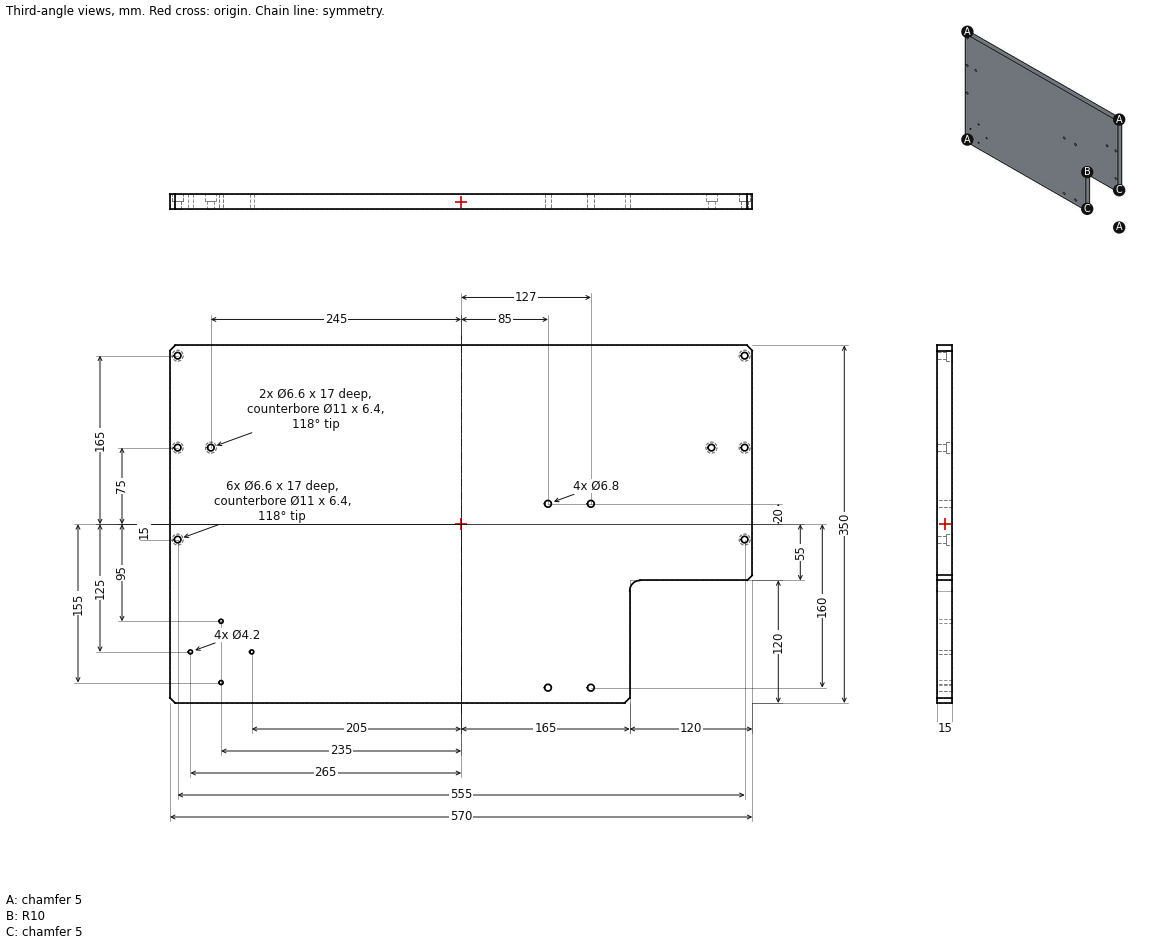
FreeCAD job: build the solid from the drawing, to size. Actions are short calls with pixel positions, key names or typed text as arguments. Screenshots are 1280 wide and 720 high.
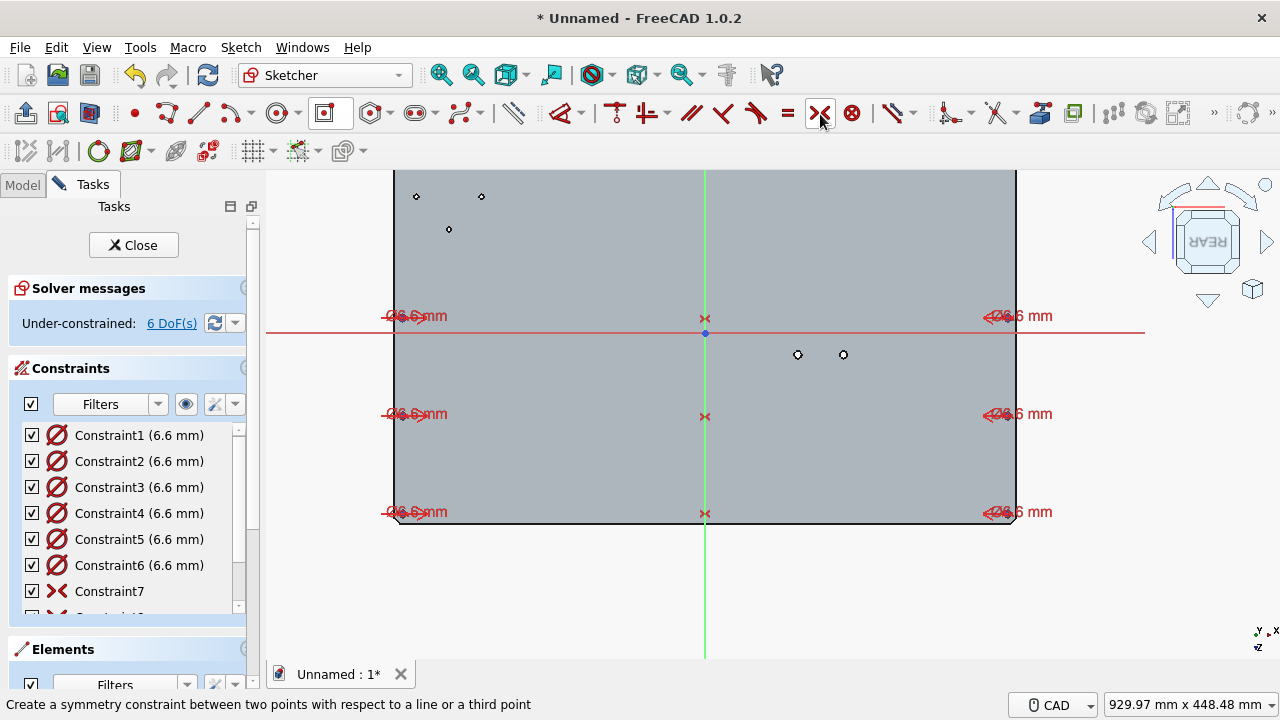
click(560, 114)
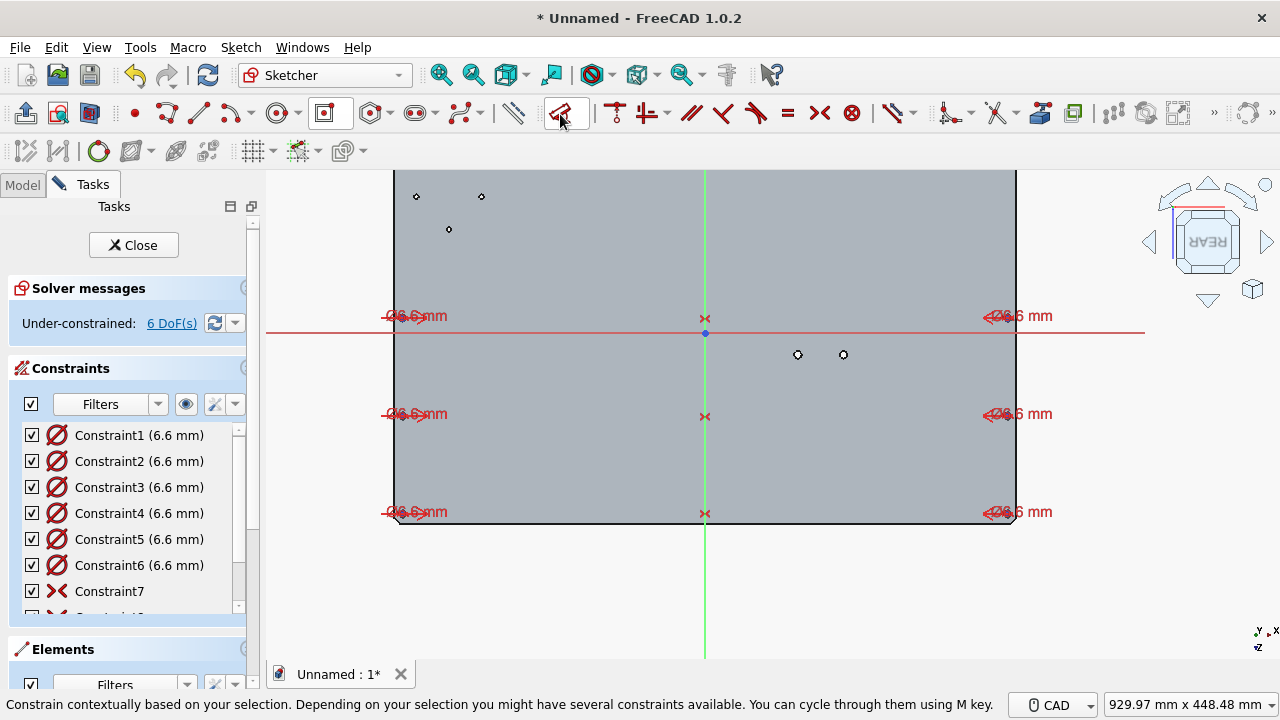
scroll(402, 318, up, 5)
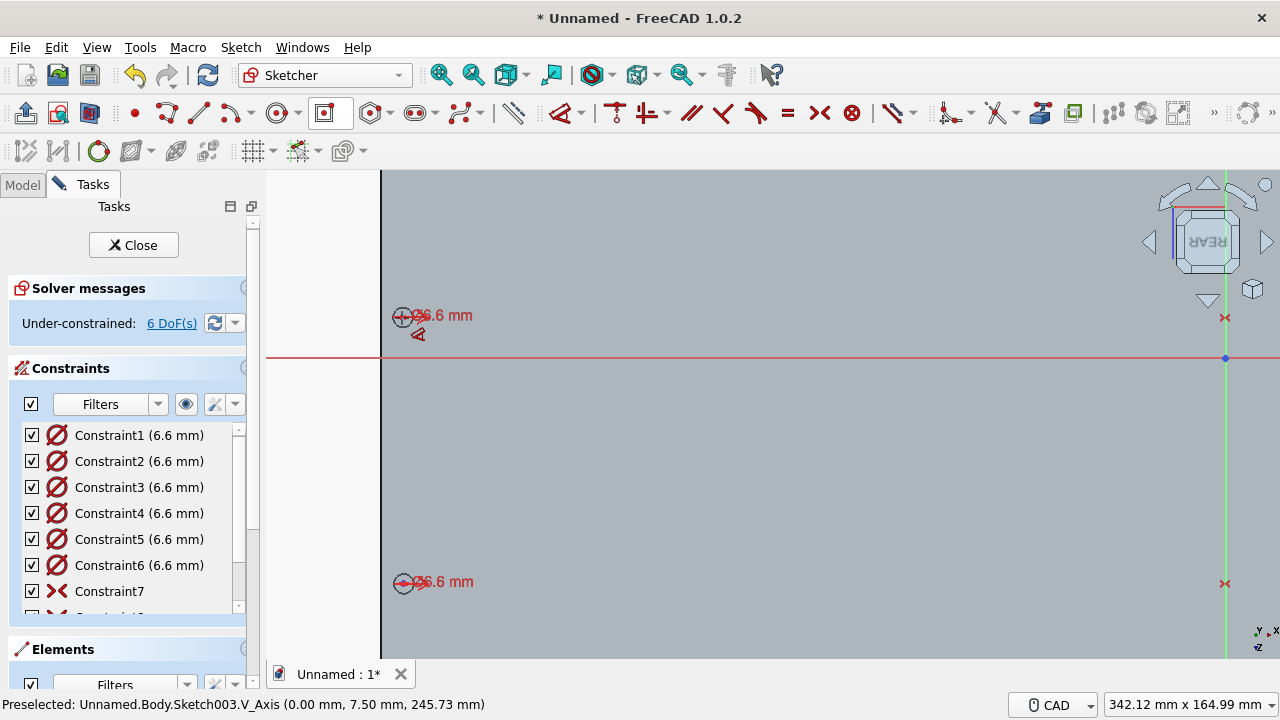
click(403, 317)
click(369, 338)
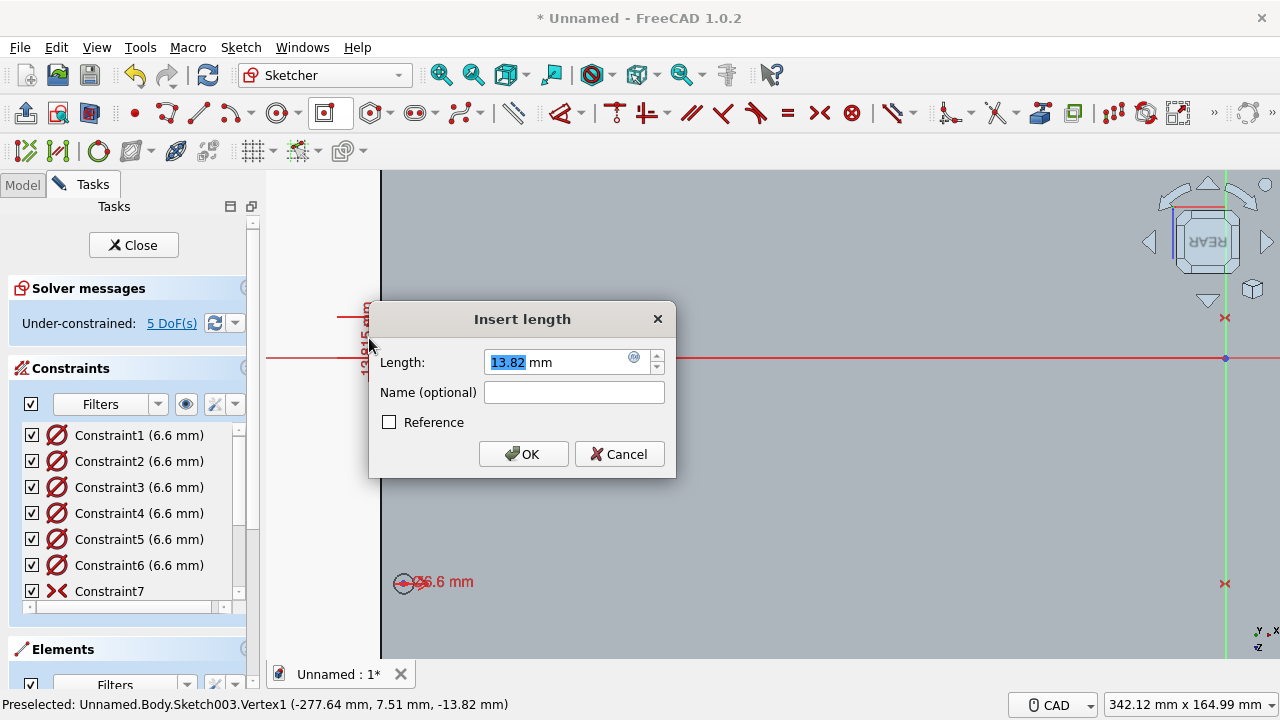
text(15)
key(Return)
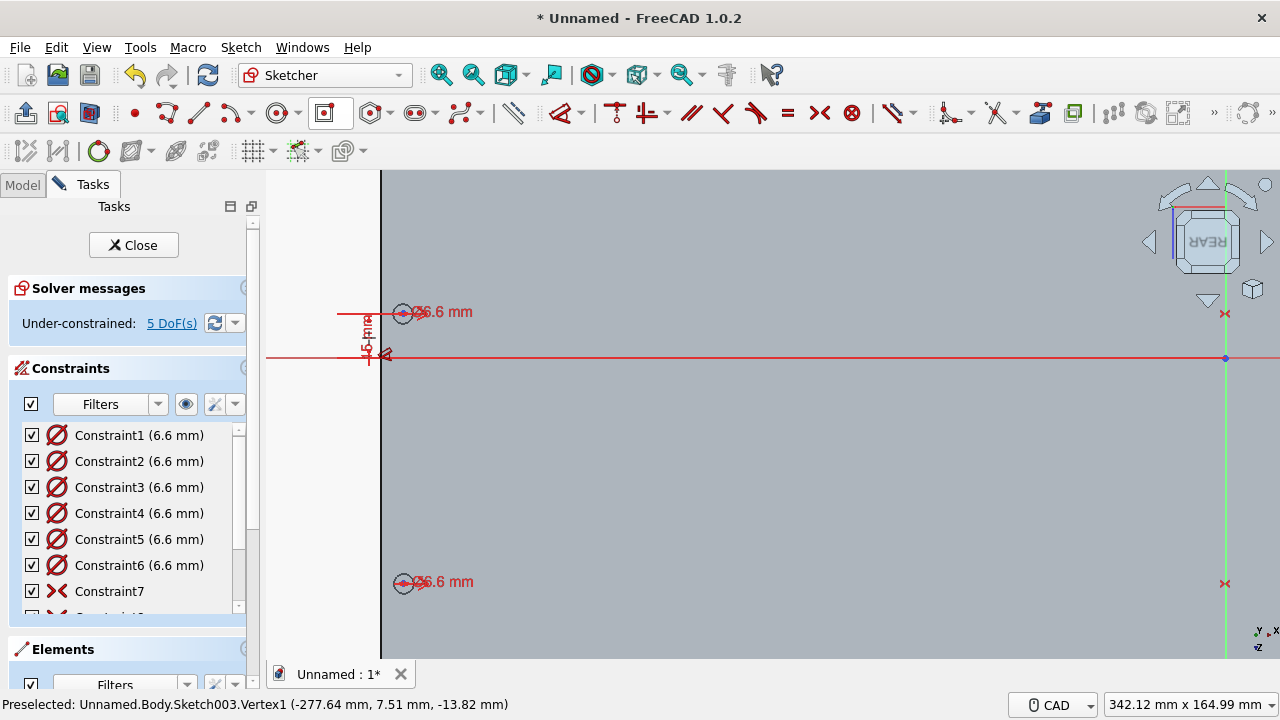
click(404, 584)
click(370, 471)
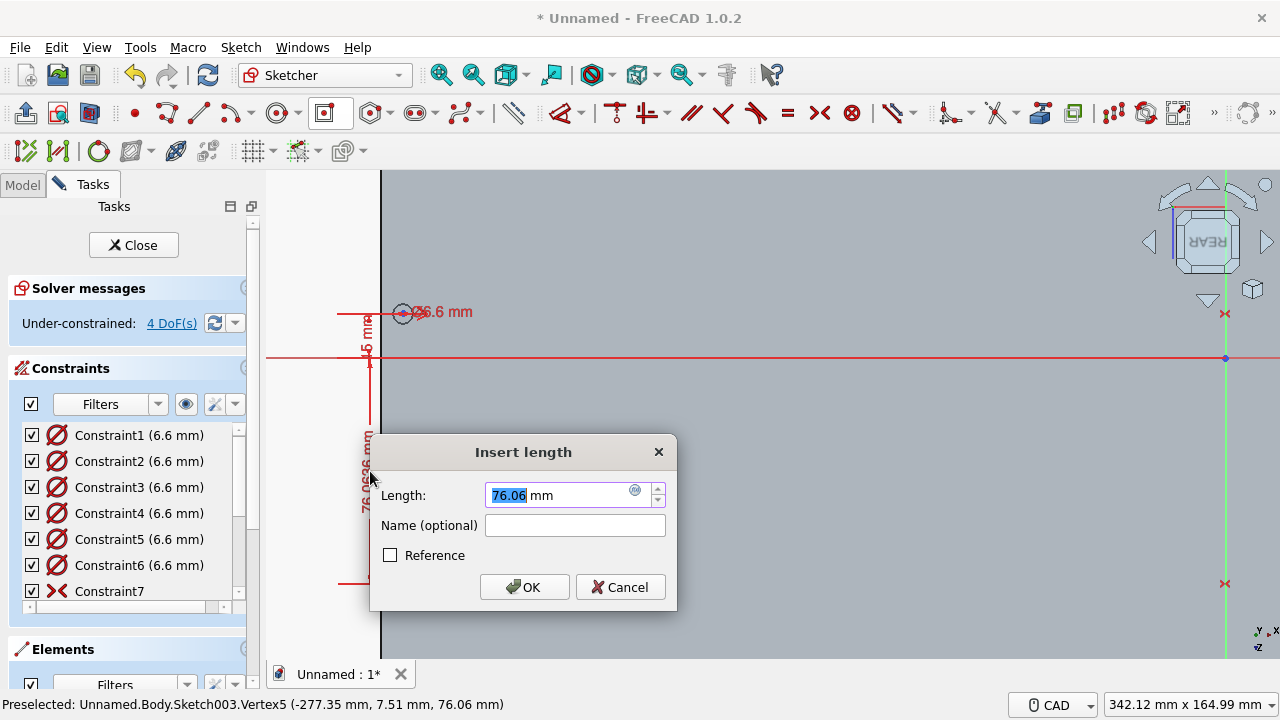
text(75)
key(Return)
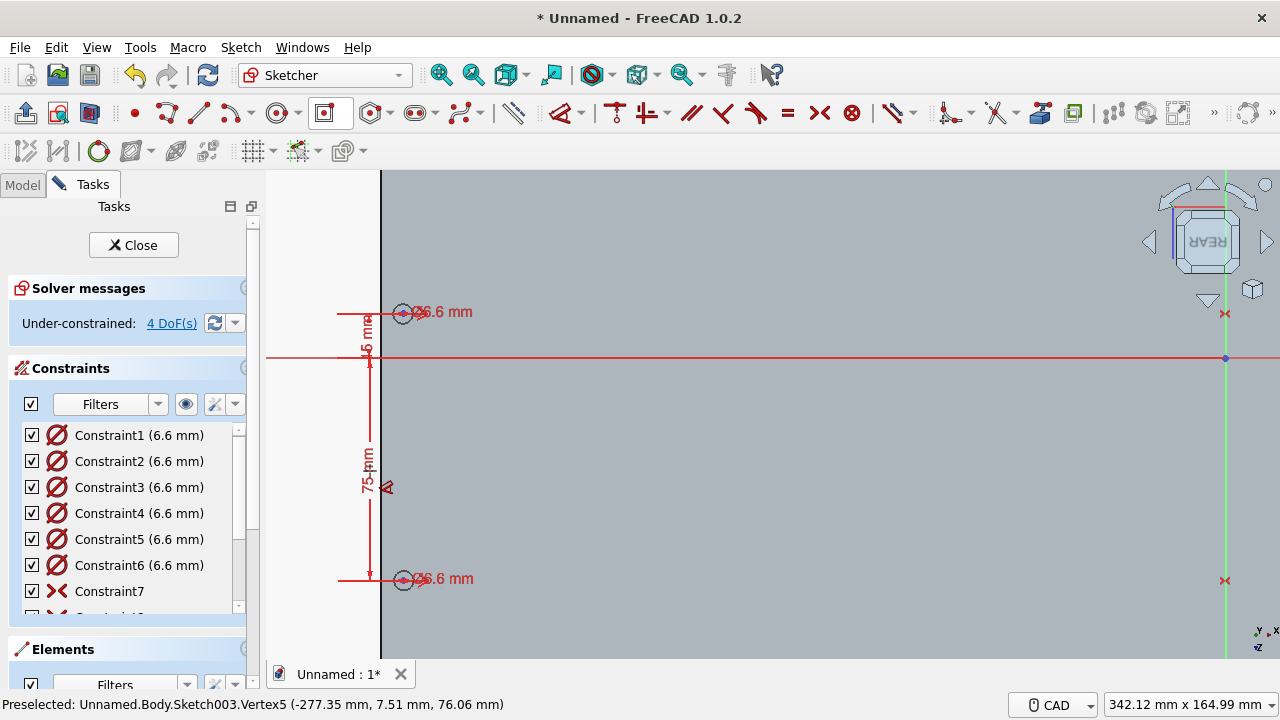
scroll(401, 318, down, 5)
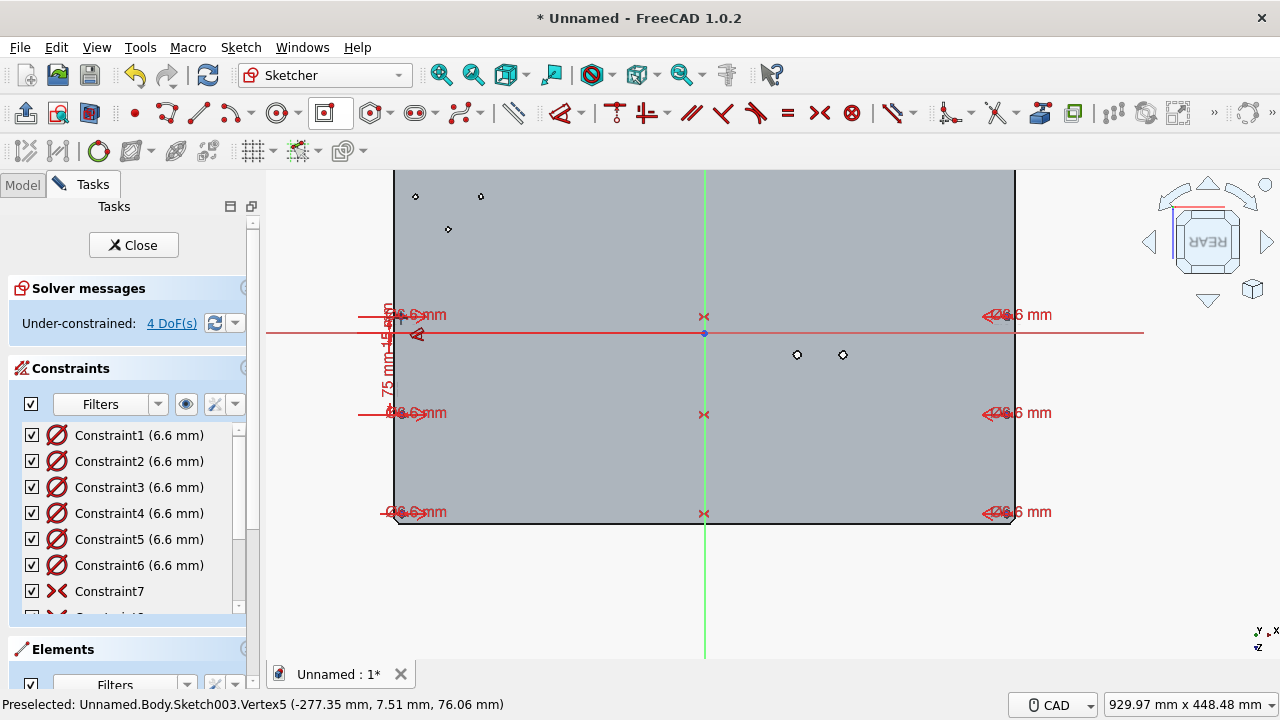
click(402, 514)
click(368, 424)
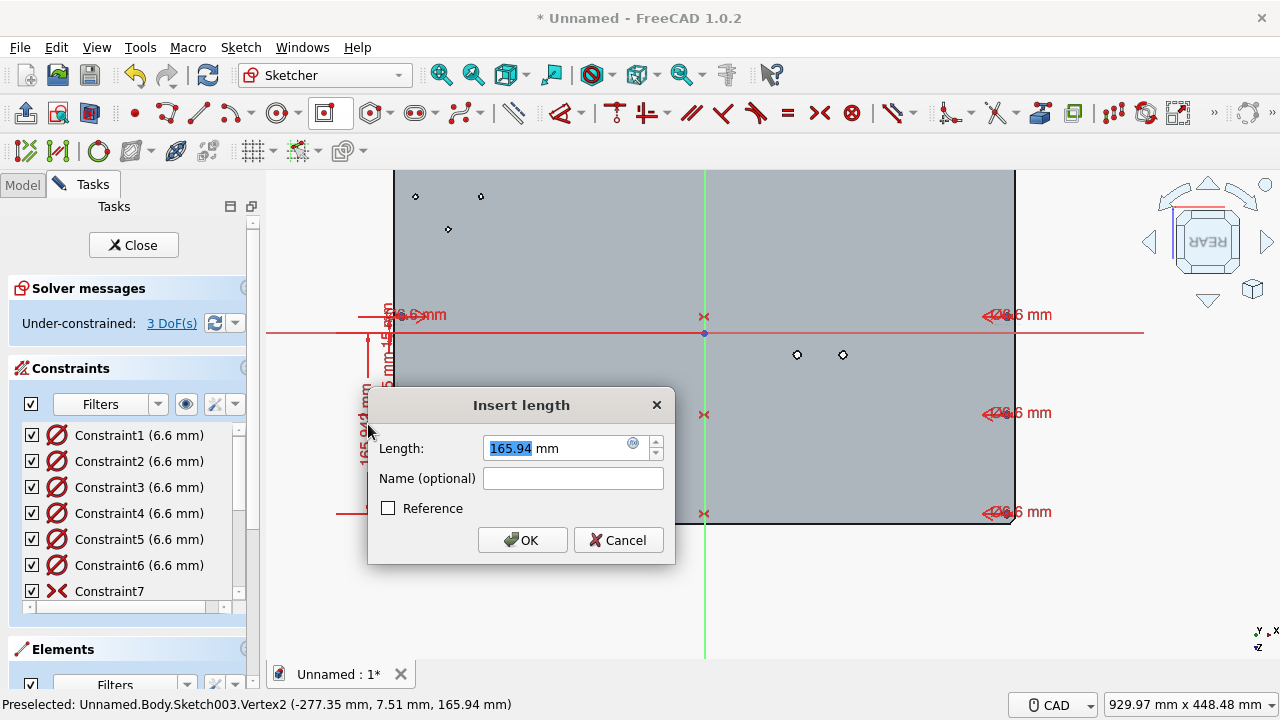
text(165)
key(Return)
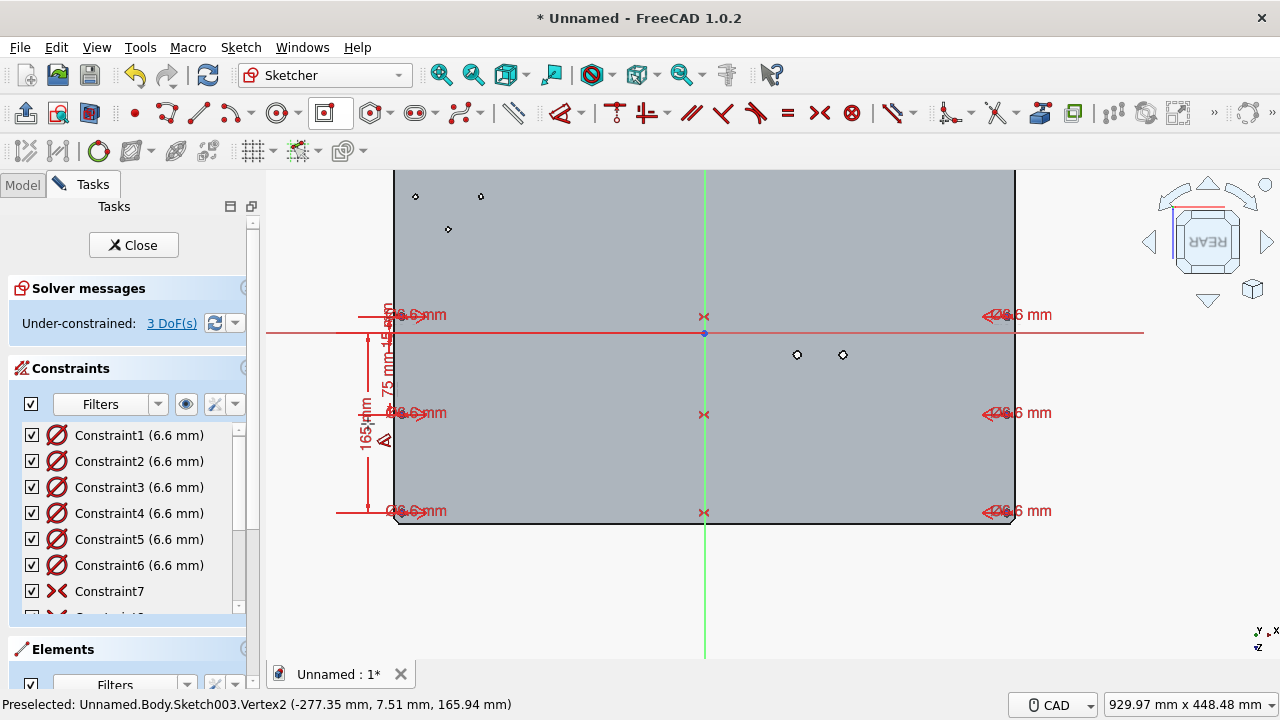
click(402, 317)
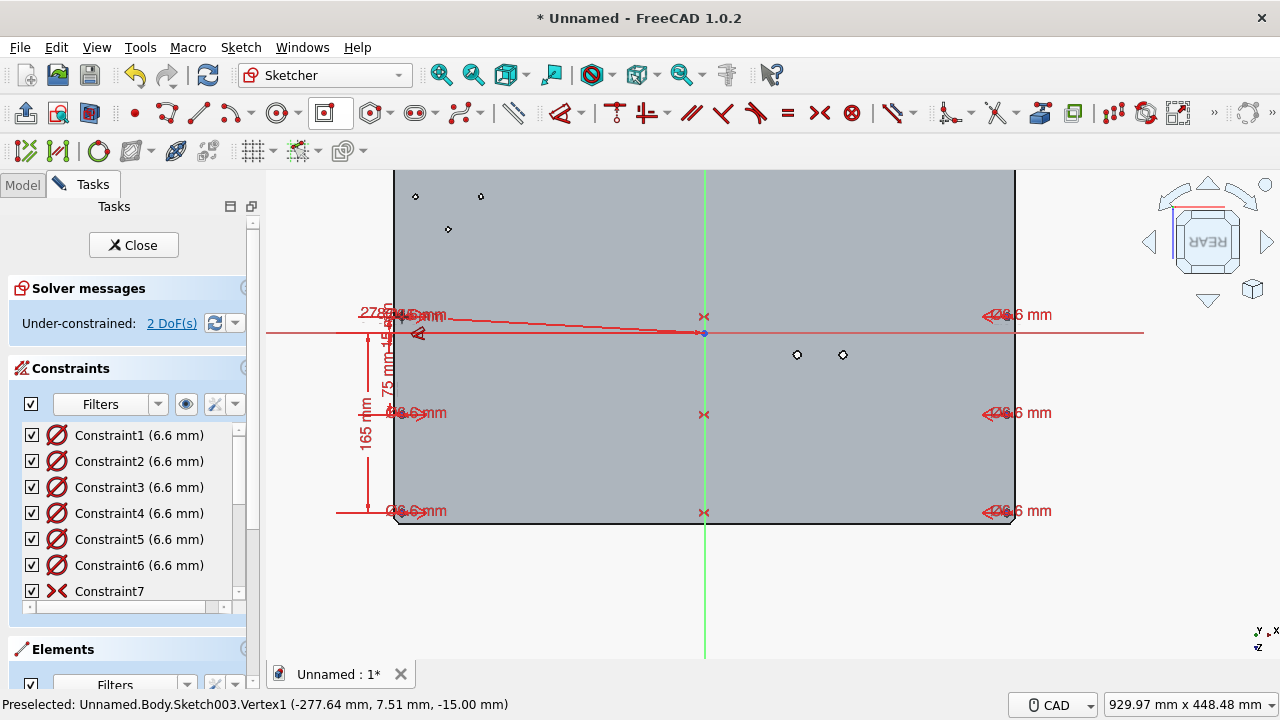
click(1007, 317)
click(565, 283)